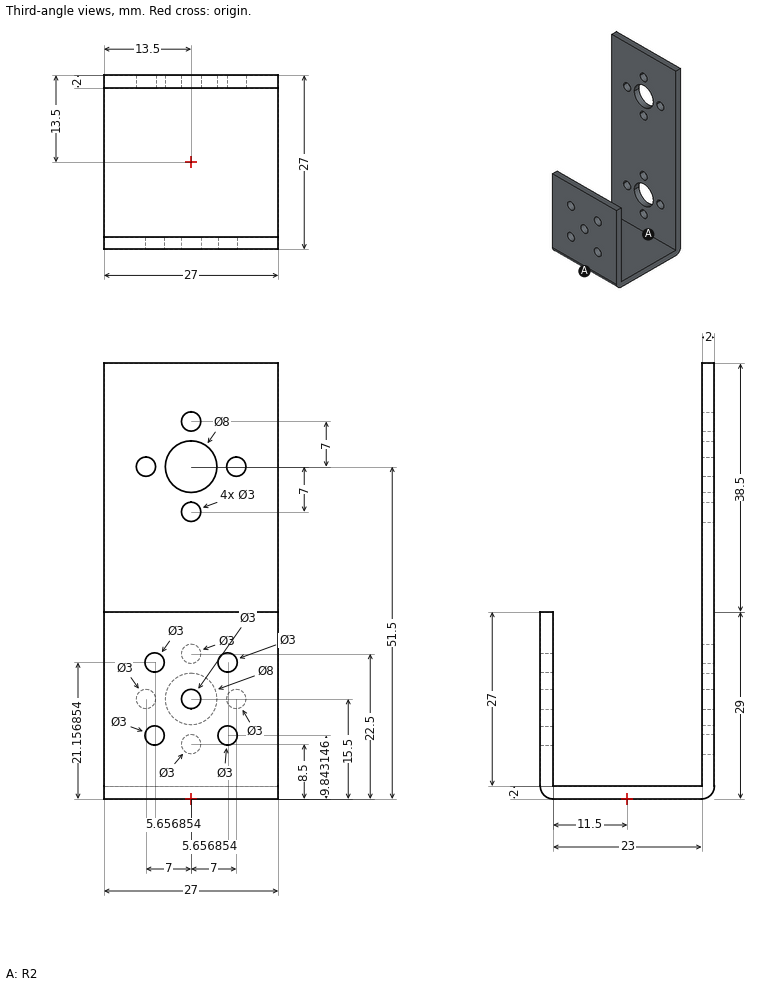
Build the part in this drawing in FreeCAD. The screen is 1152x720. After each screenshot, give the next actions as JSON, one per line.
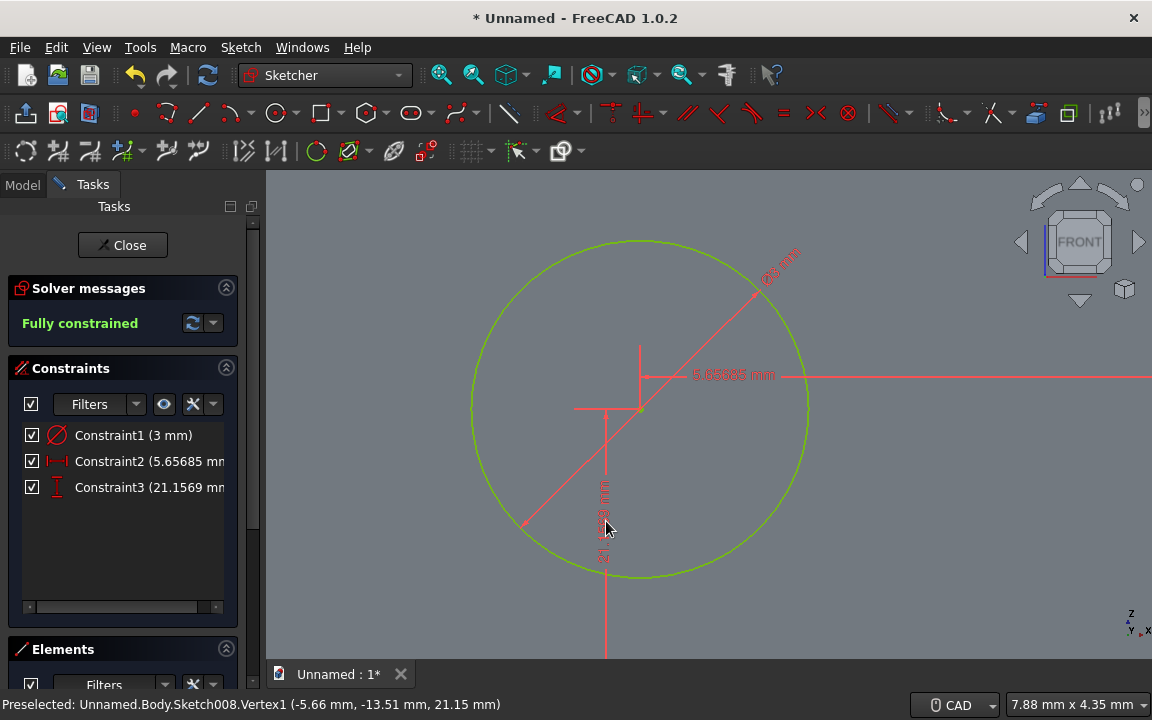
{"action": "left_click", "coordinate": [123, 245]}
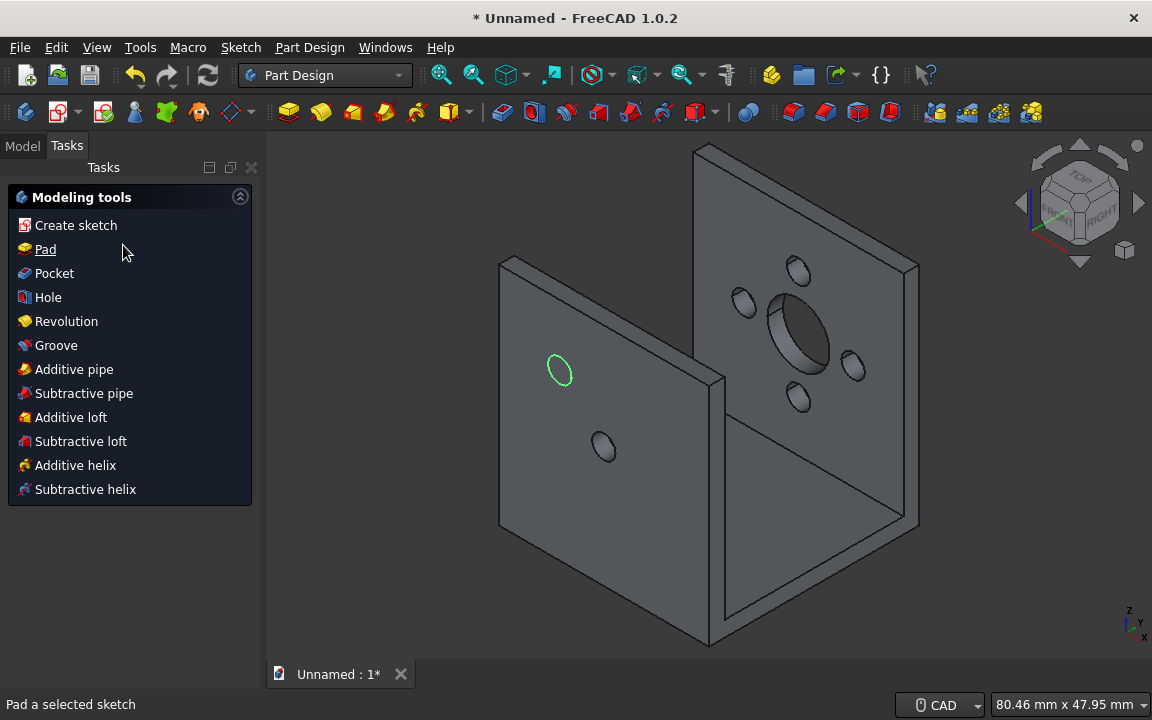
{"action": "left_click", "coordinate": [504, 112]}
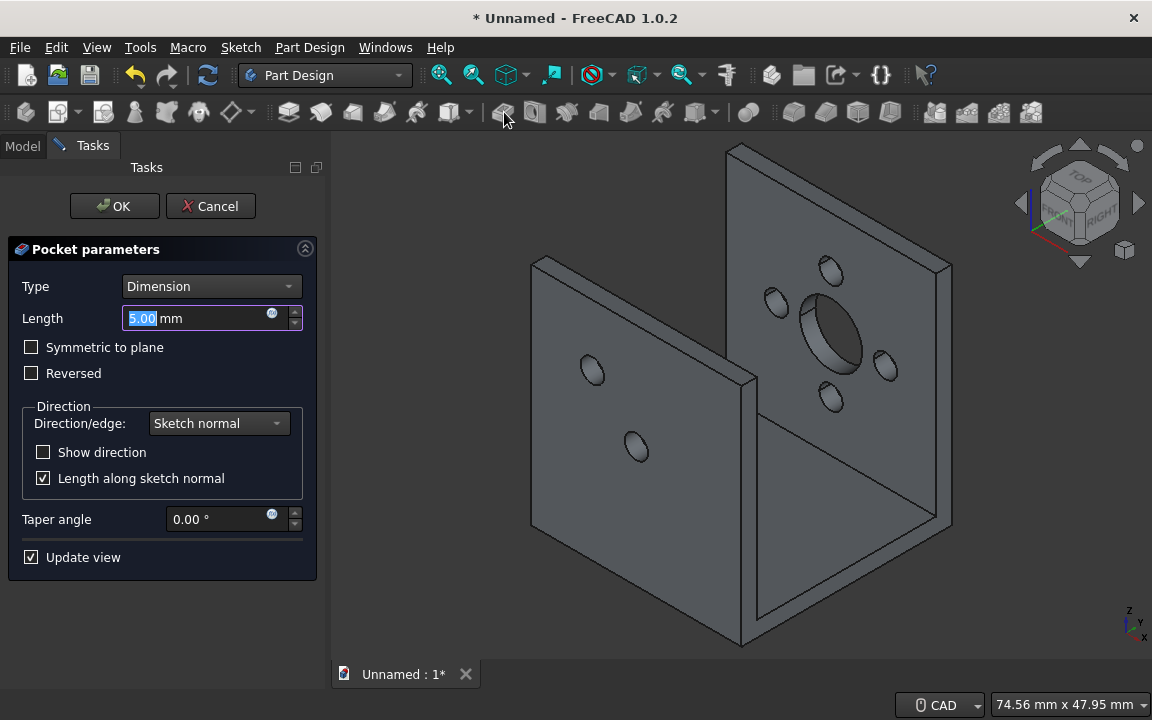
{"action": "left_click", "coordinate": [212, 286]}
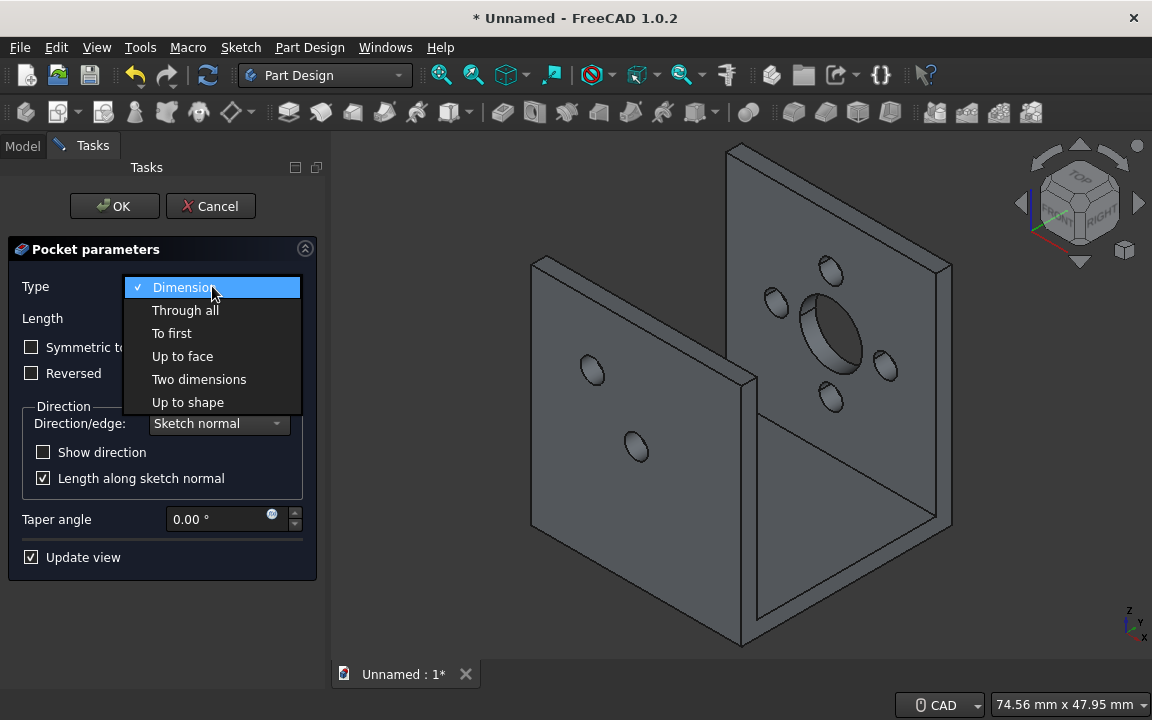
{"action": "left_click", "coordinate": [212, 334]}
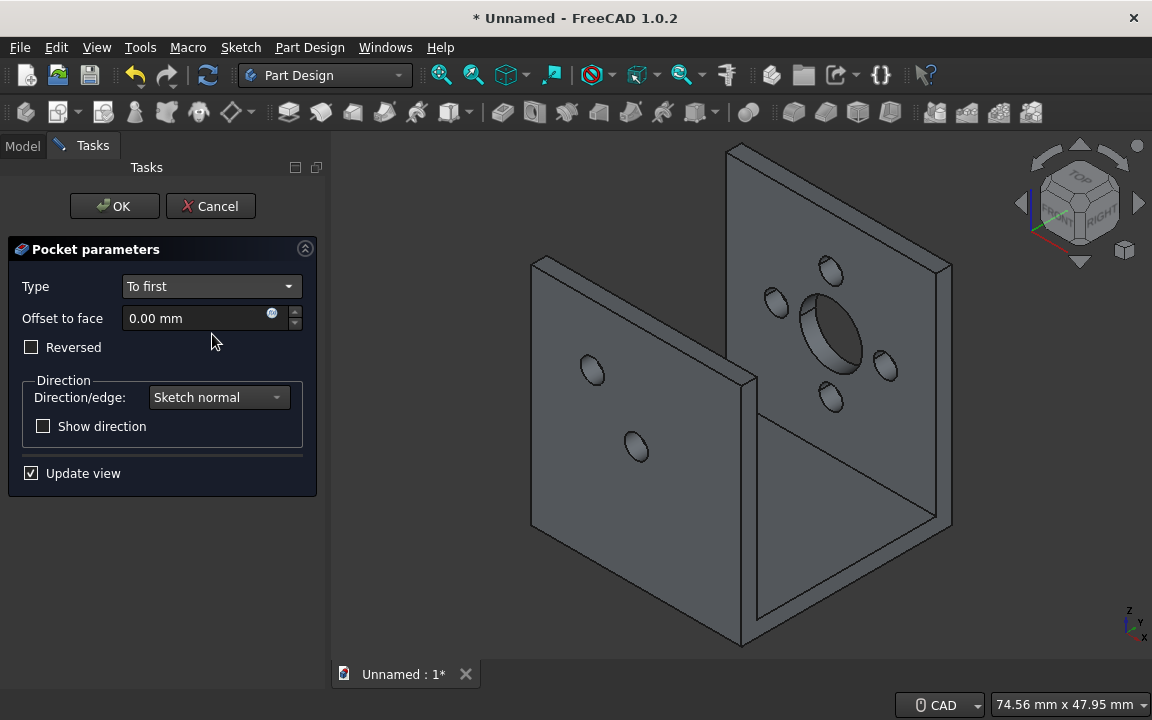
{"action": "left_click", "coordinate": [115, 206]}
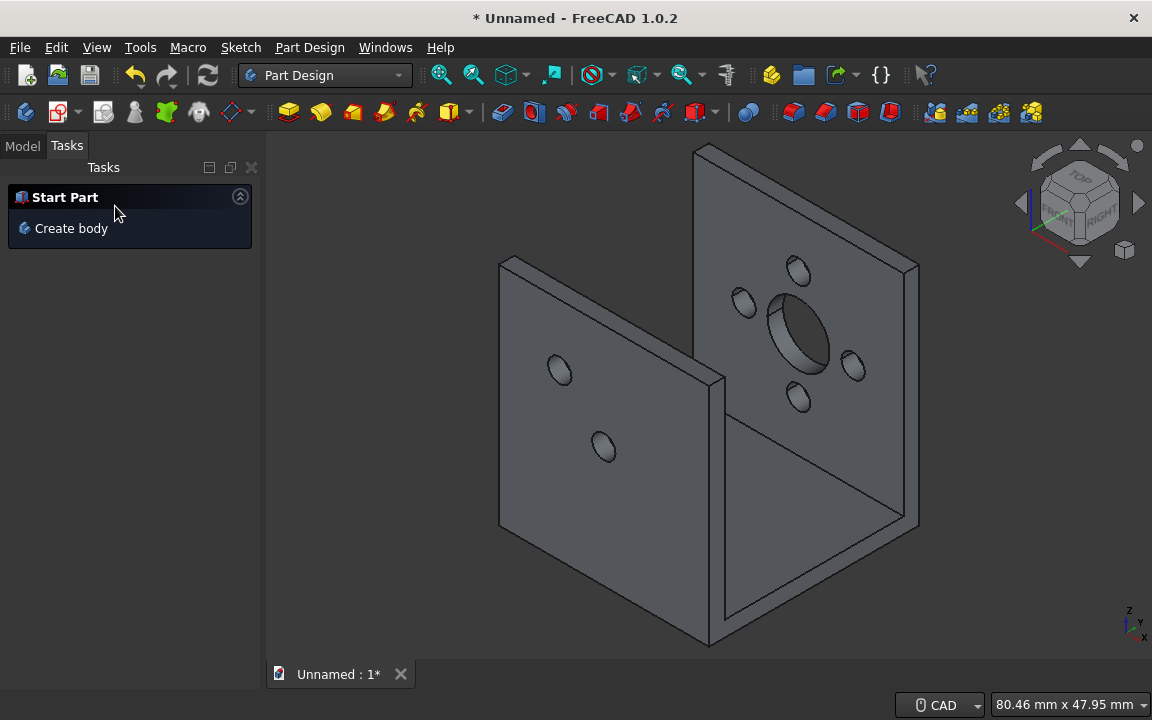
{"action": "left_click", "coordinate": [634, 398]}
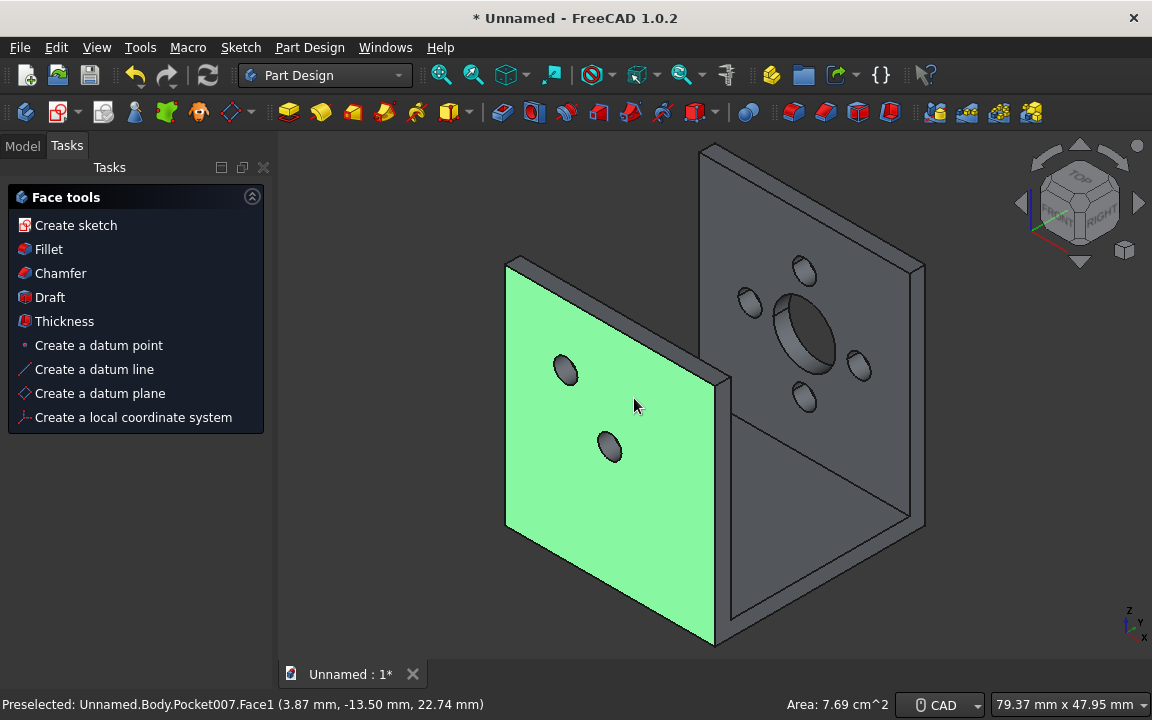
{"action": "left_click", "coordinate": [58, 112]}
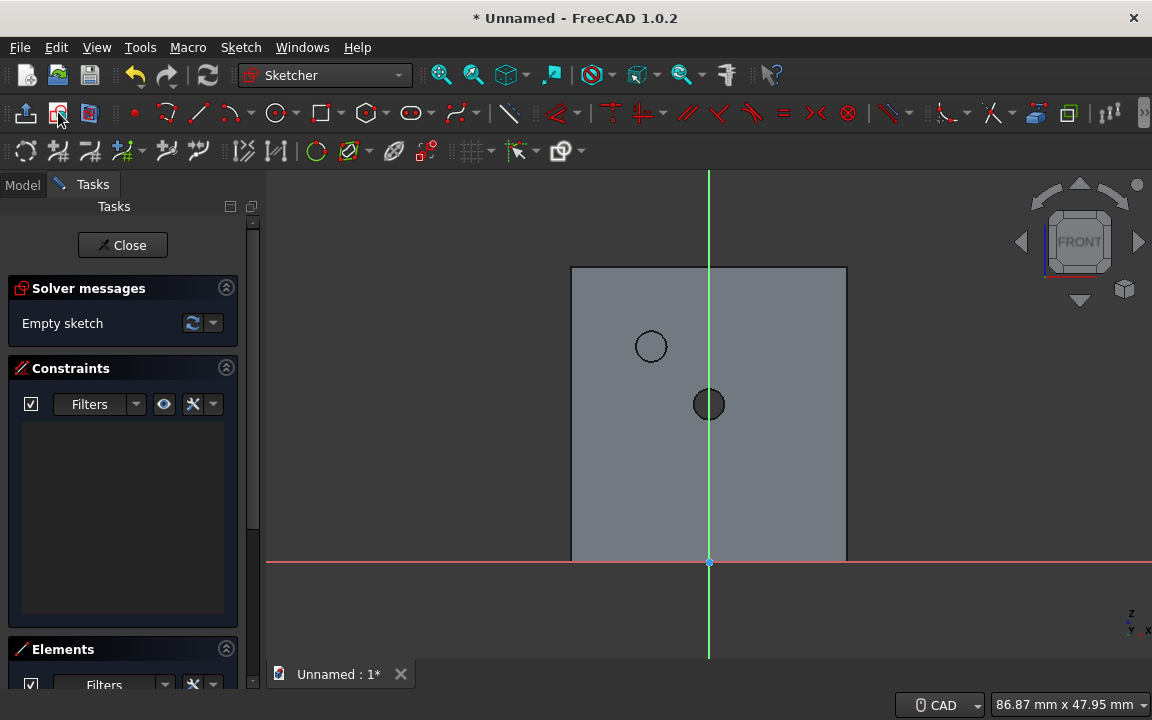
{"action": "scroll", "coordinate": [779, 340], "scroll_direction": "up", "scroll_amount": 12}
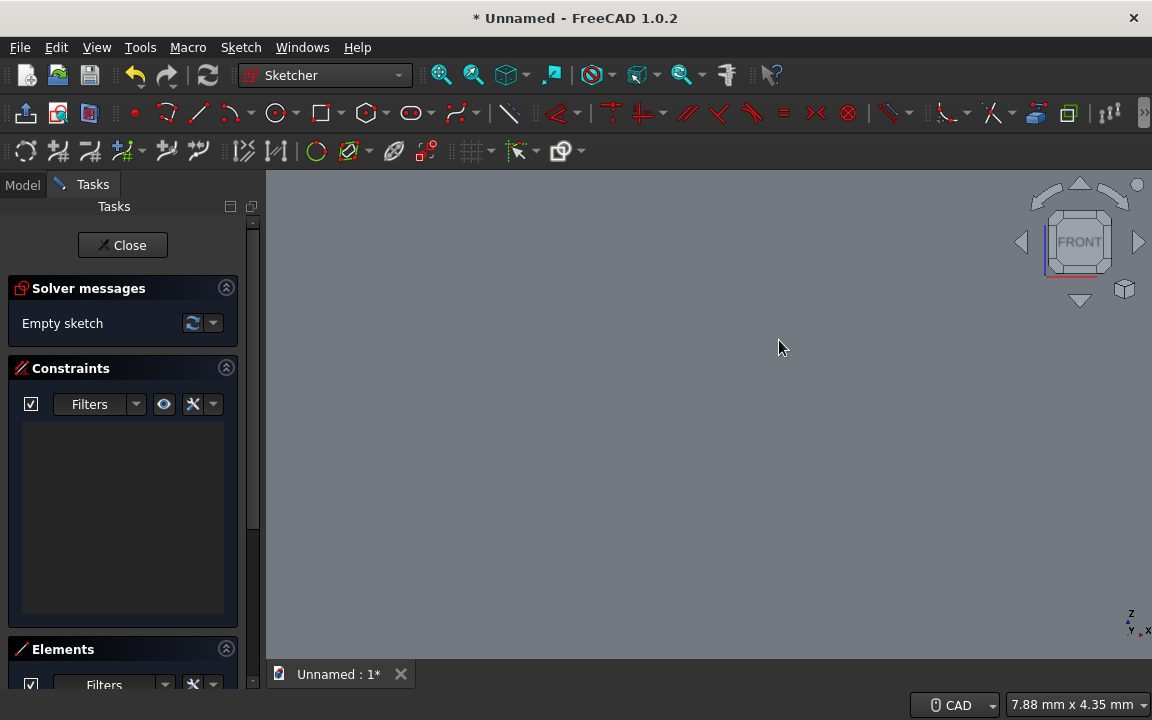
{"action": "key", "text": "g c"}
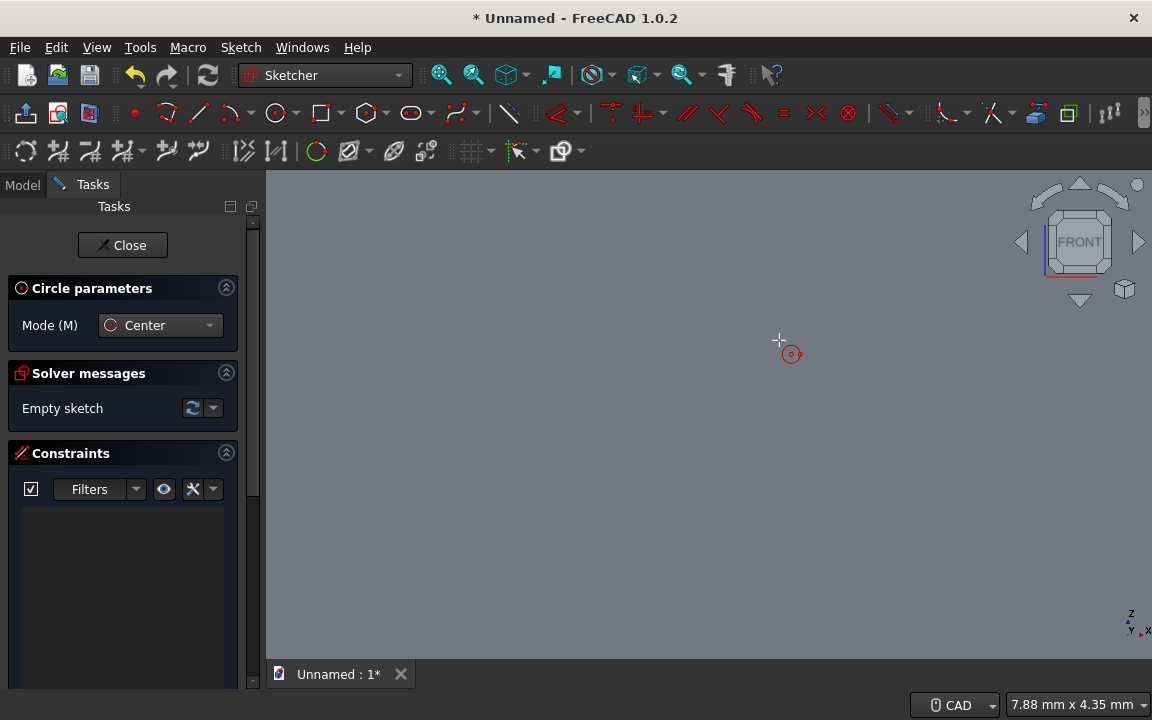
{"action": "left_click", "coordinate": [638, 409]}
{"action": "left_click", "coordinate": [757, 290]}
{"action": "key", "text": "Escape"}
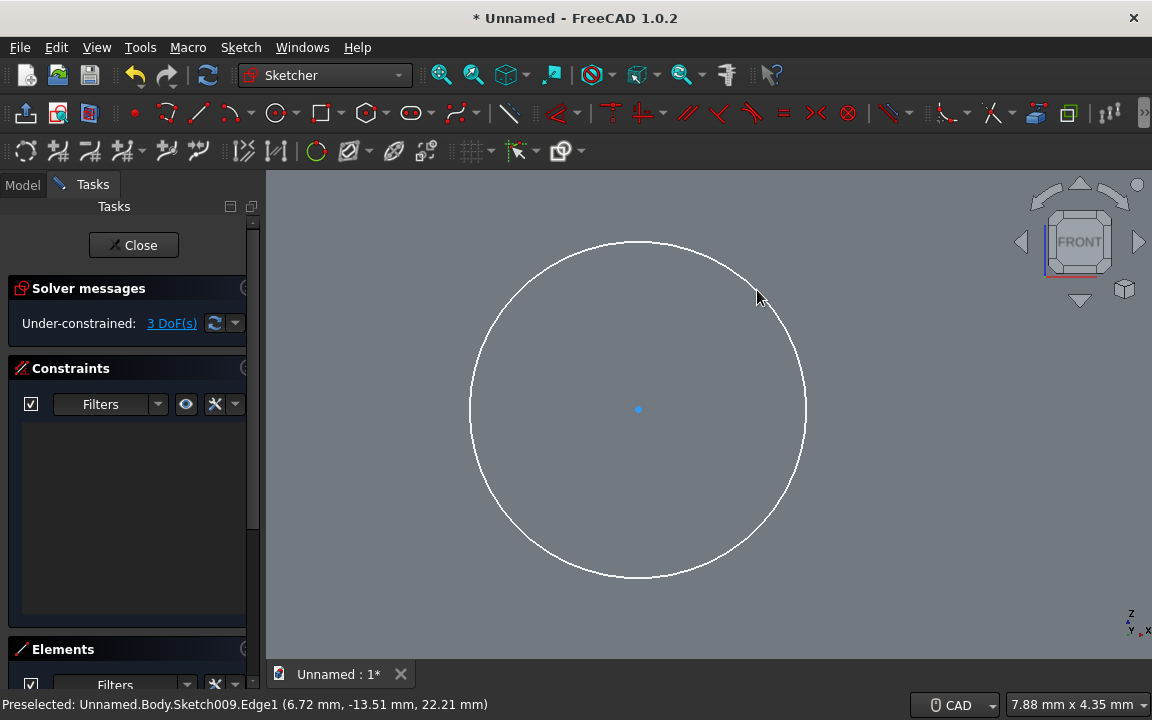
{"action": "key", "text": "d"}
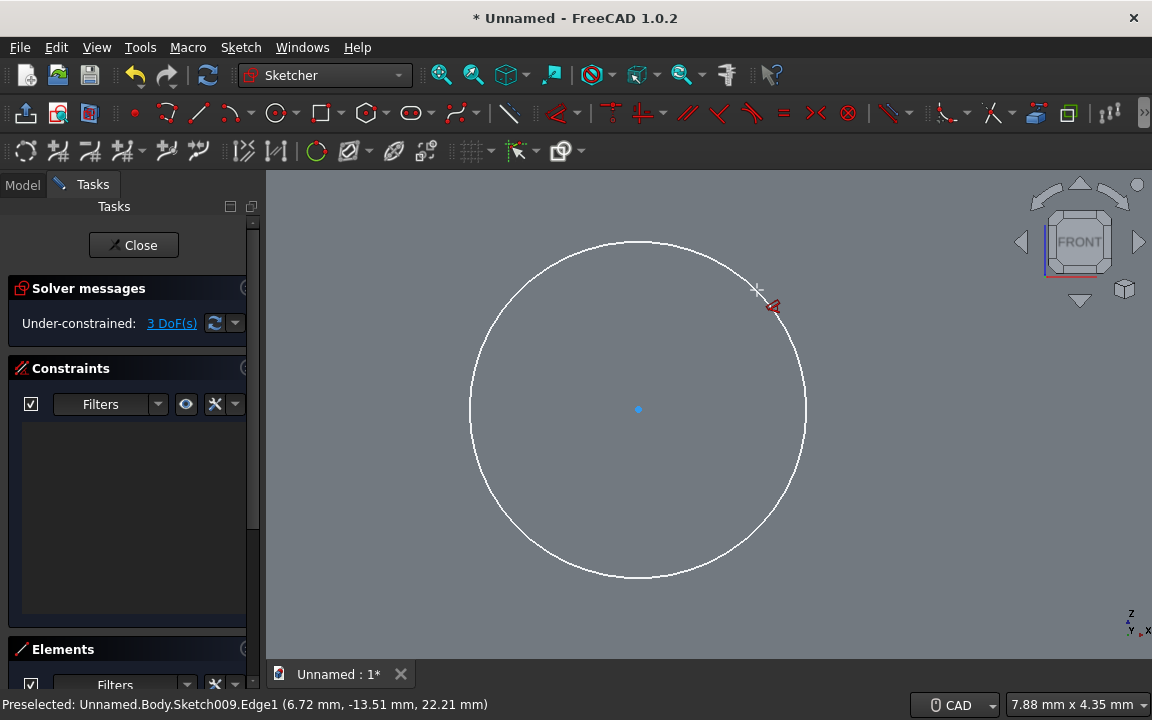
{"action": "left_click", "coordinate": [757, 291]}
{"action": "left_click", "coordinate": [780, 268]}